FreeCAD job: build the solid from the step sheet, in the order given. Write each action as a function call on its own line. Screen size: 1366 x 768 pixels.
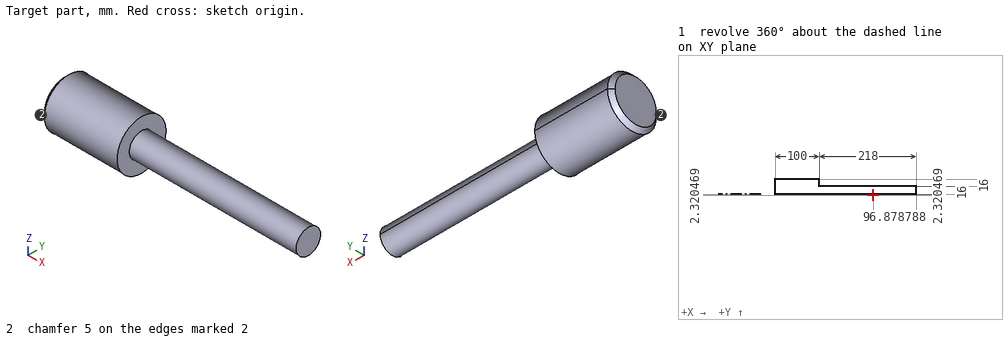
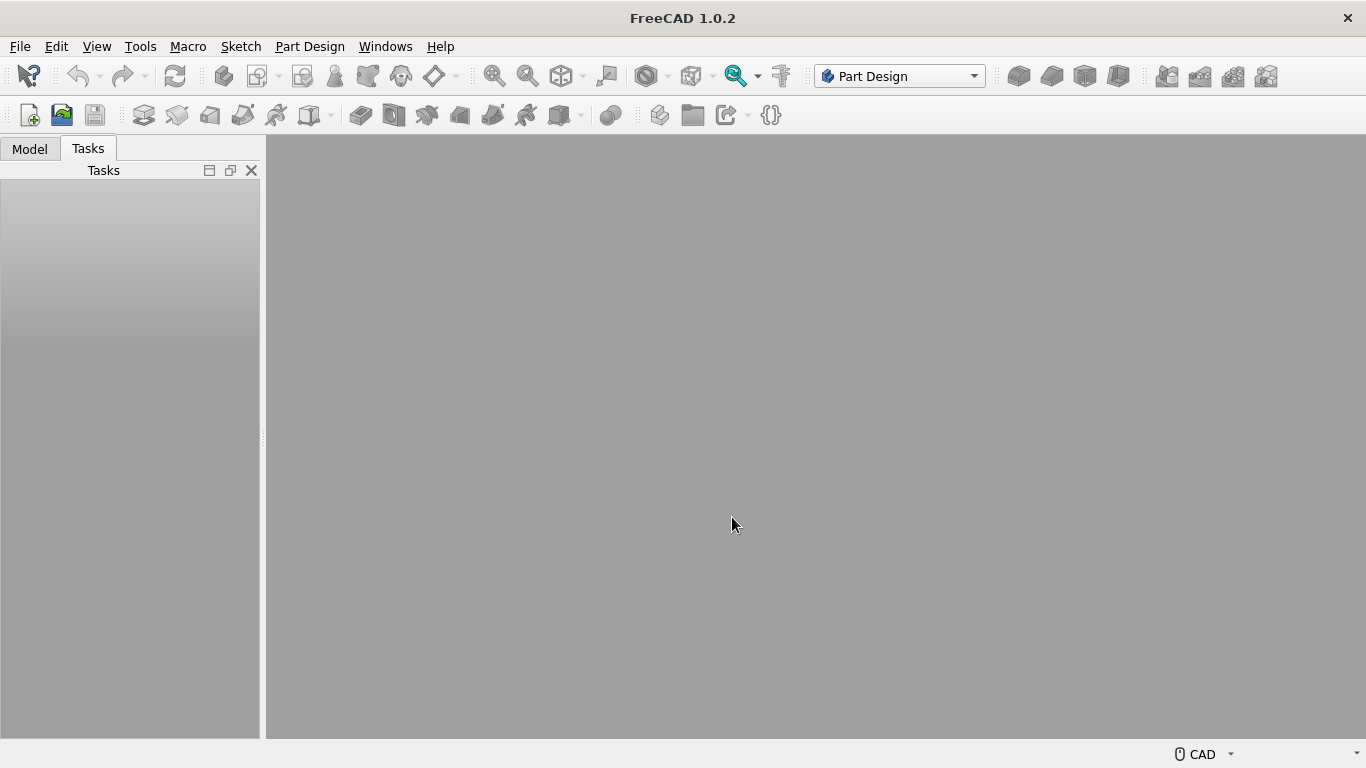
click(29, 116)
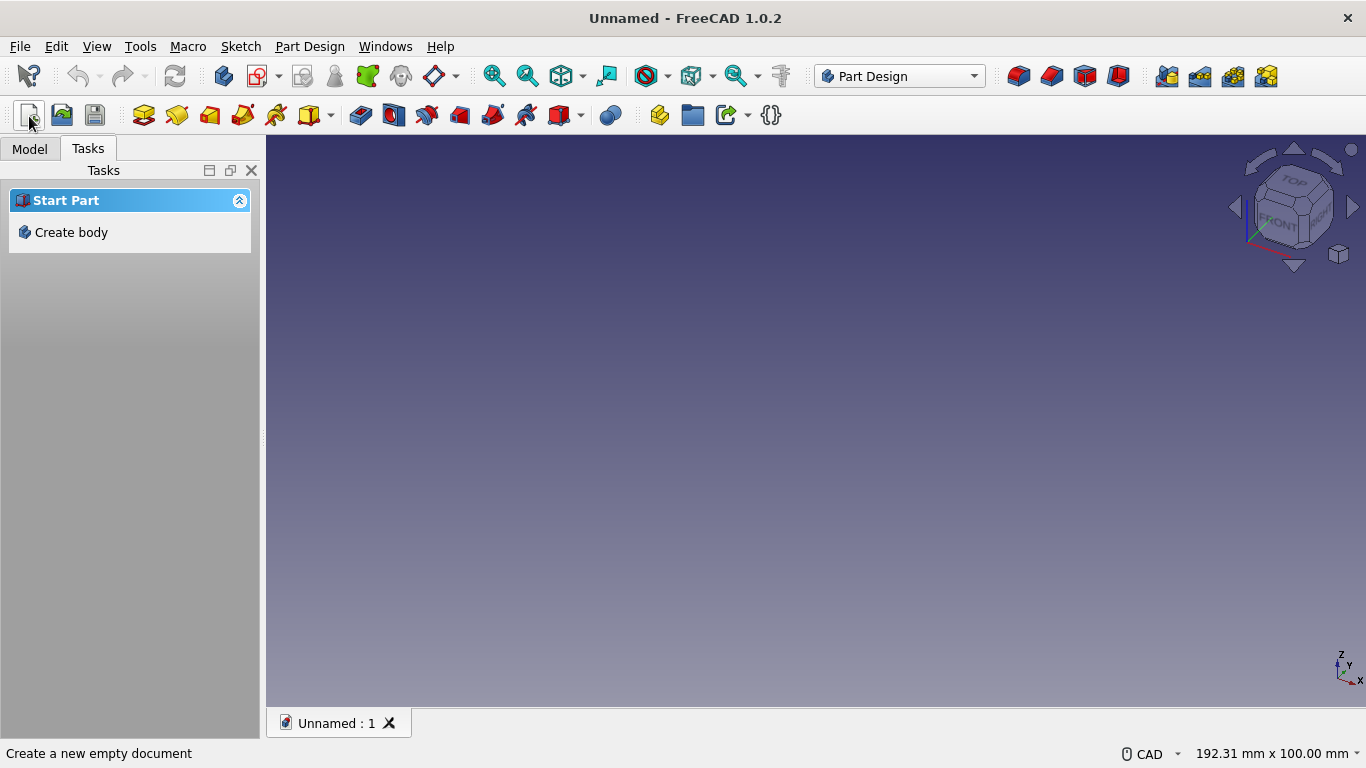
click(256, 76)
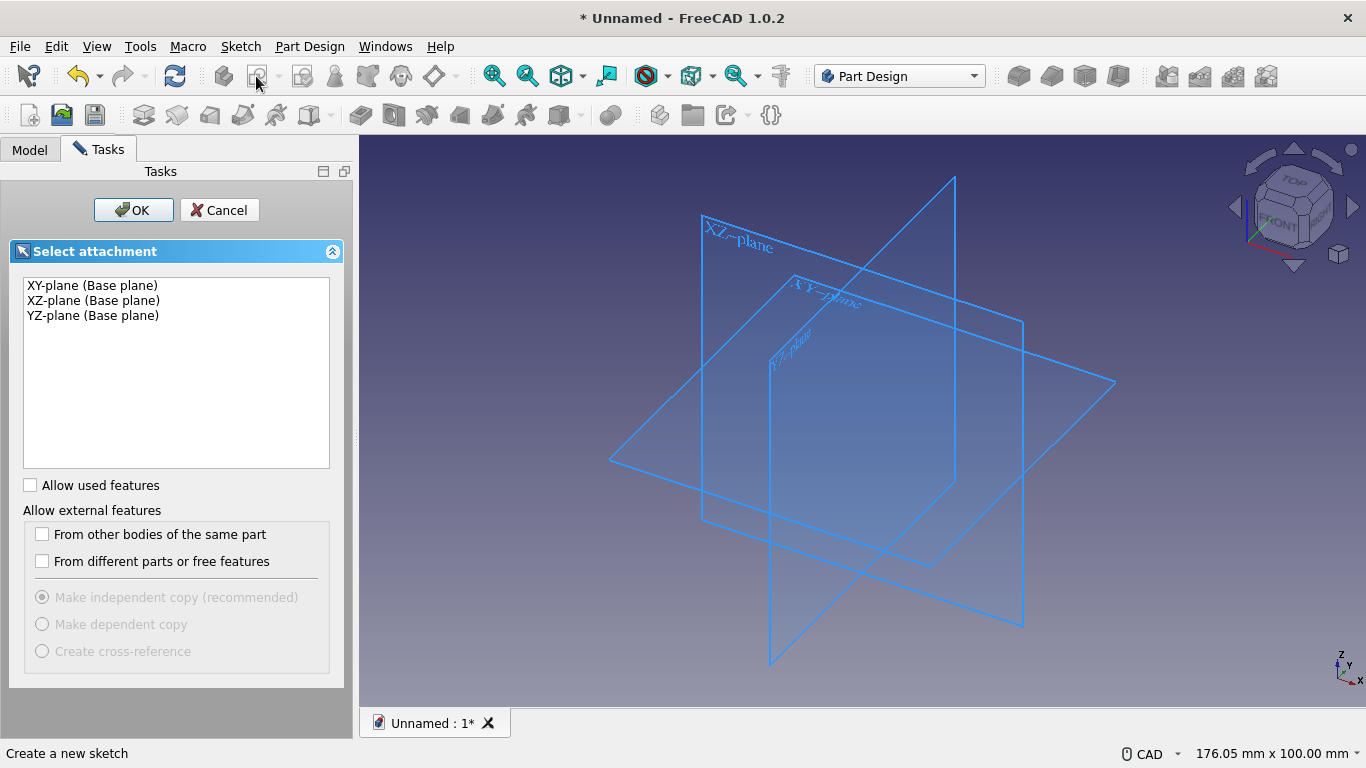
click(84, 286)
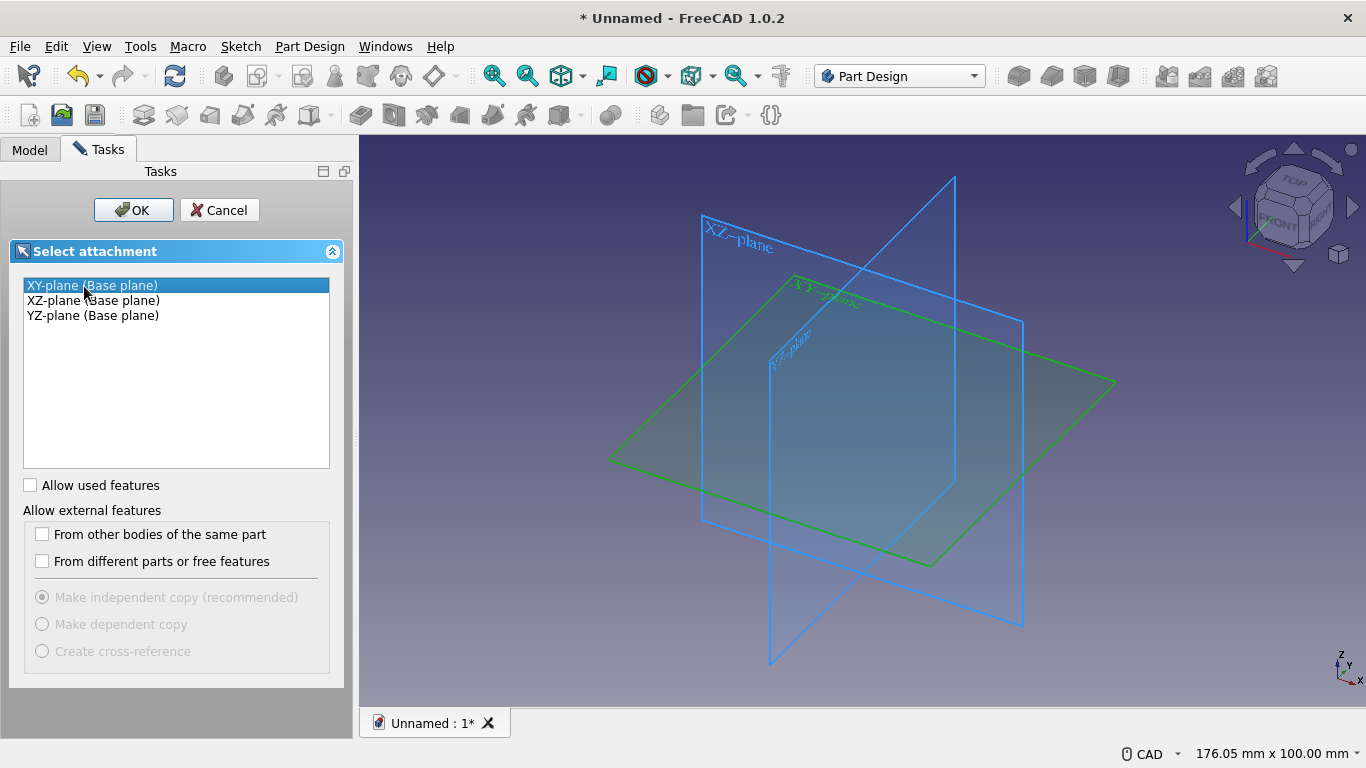
click(134, 210)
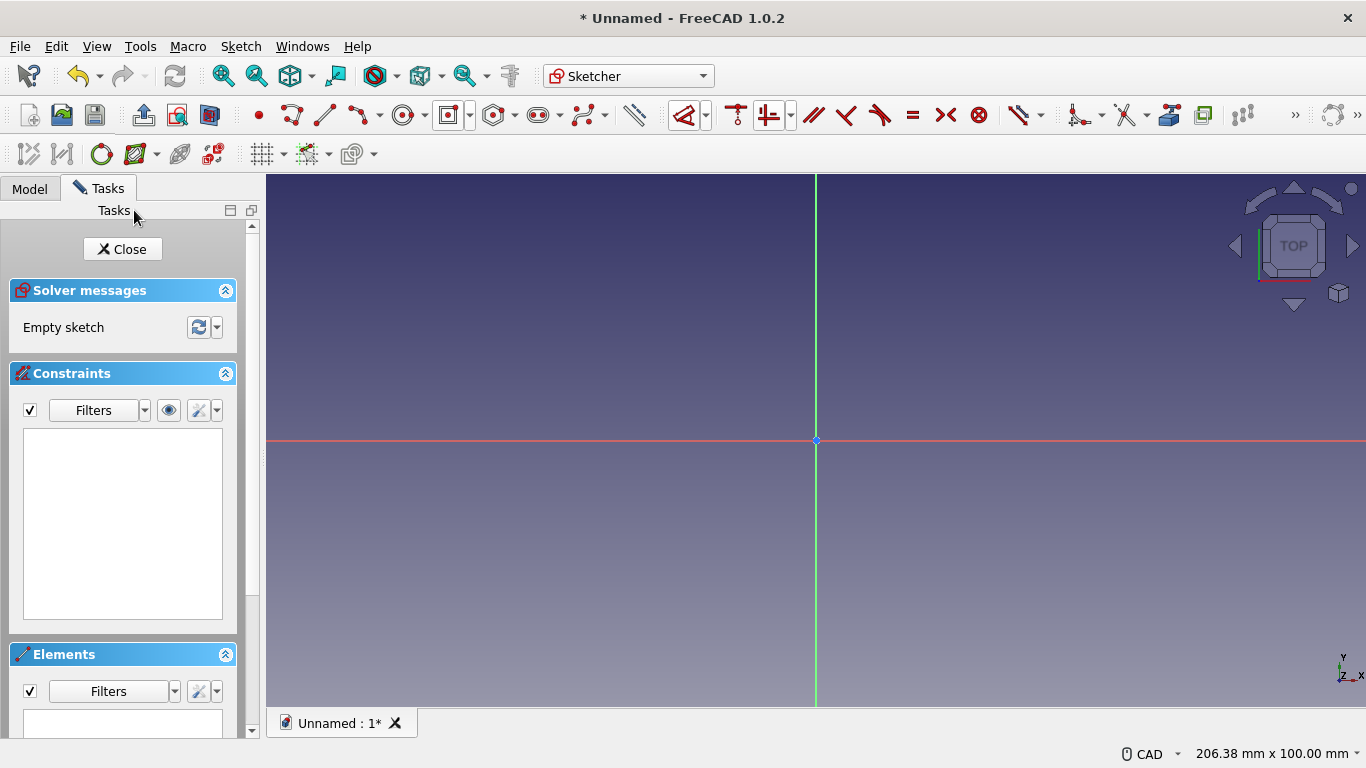
scroll(944, 470, down, 7)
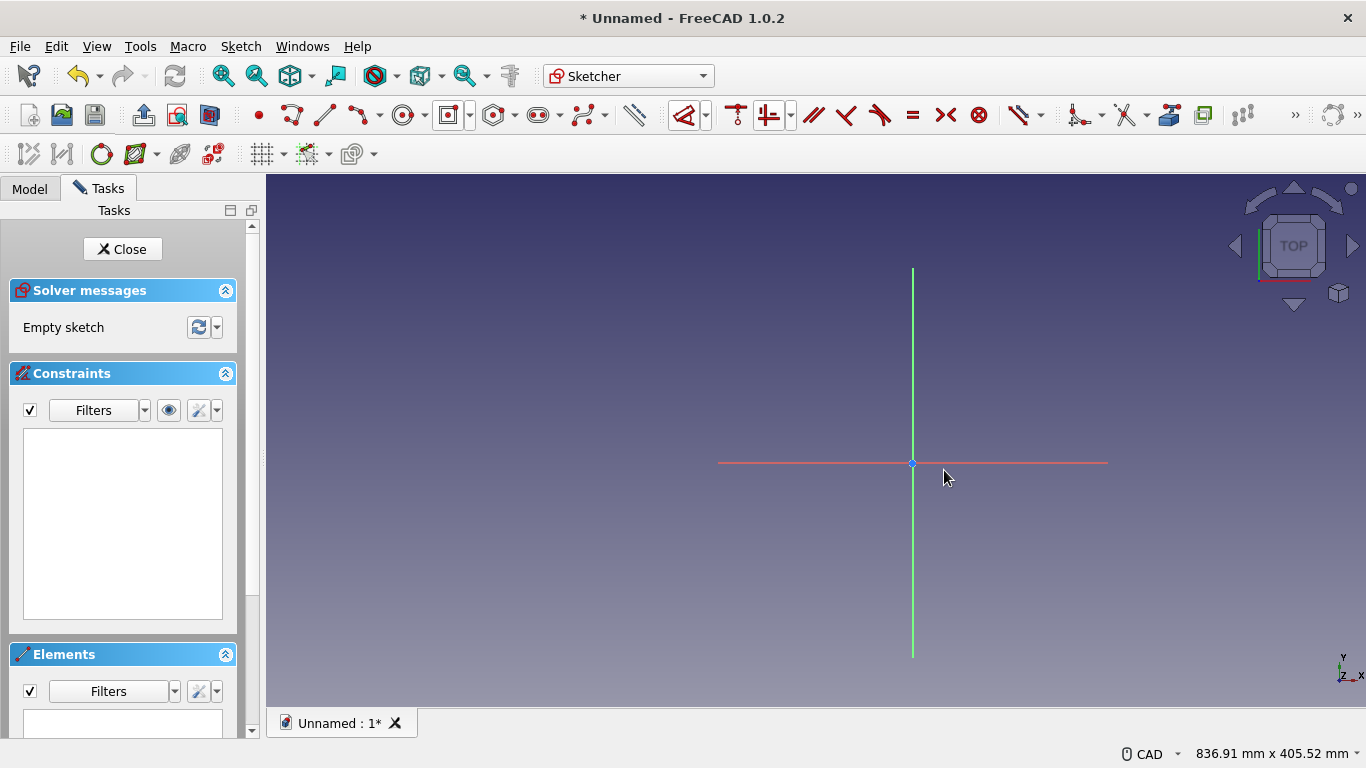
click(292, 116)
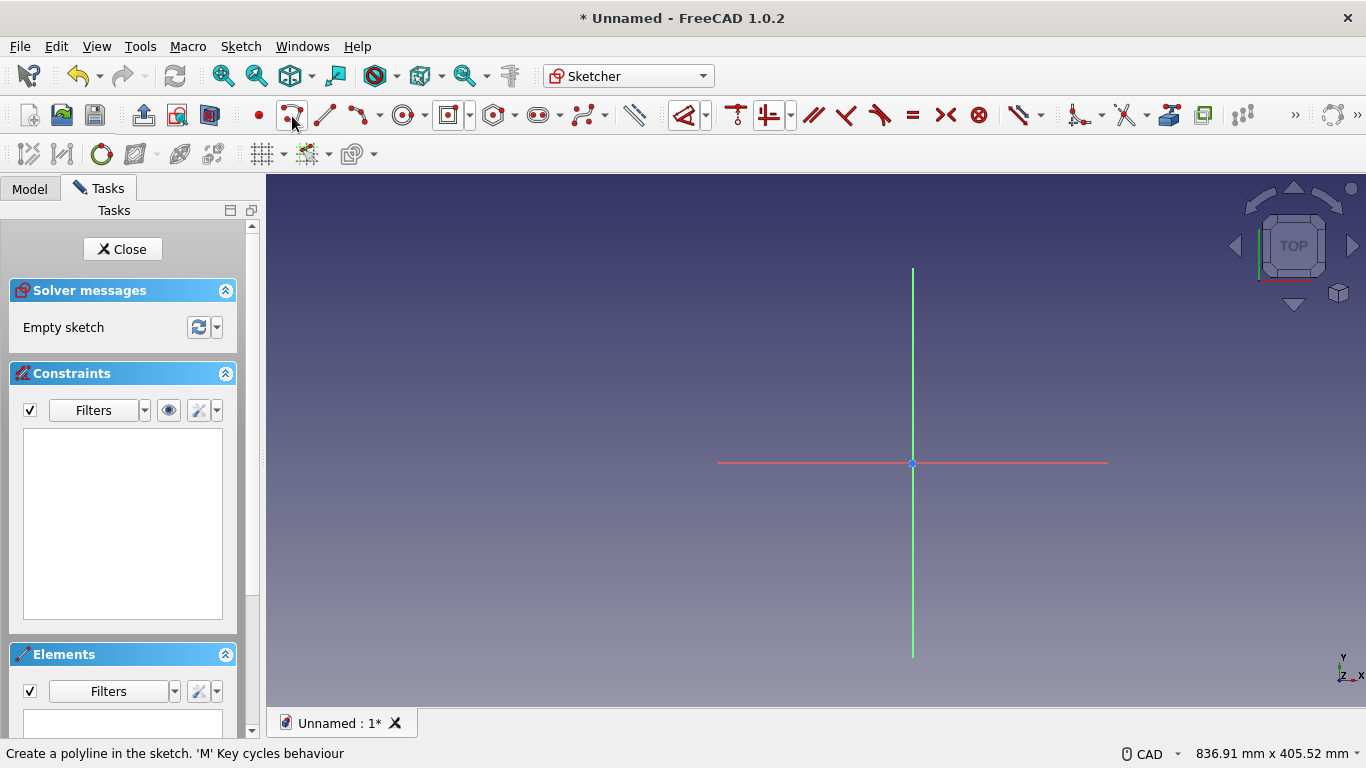
scroll(1040, 460, up, 9)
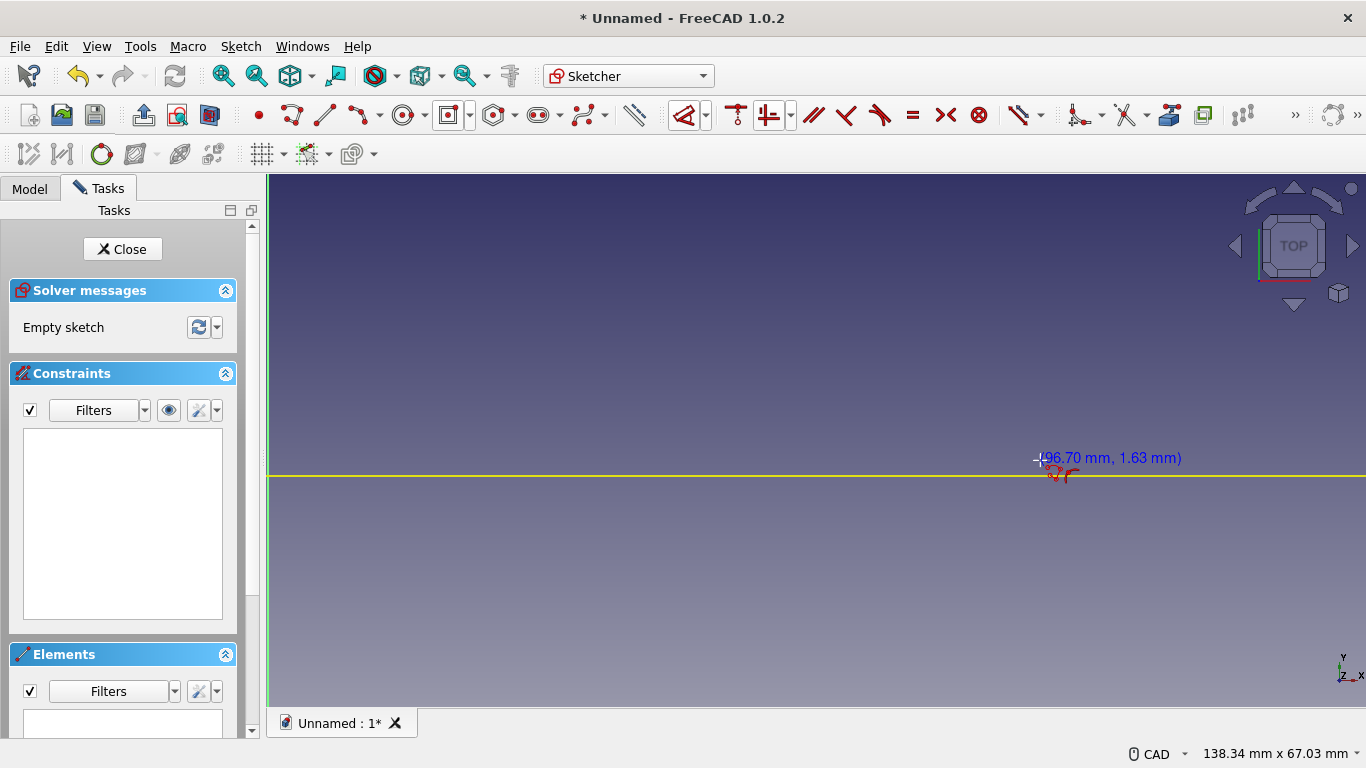
click(1038, 458)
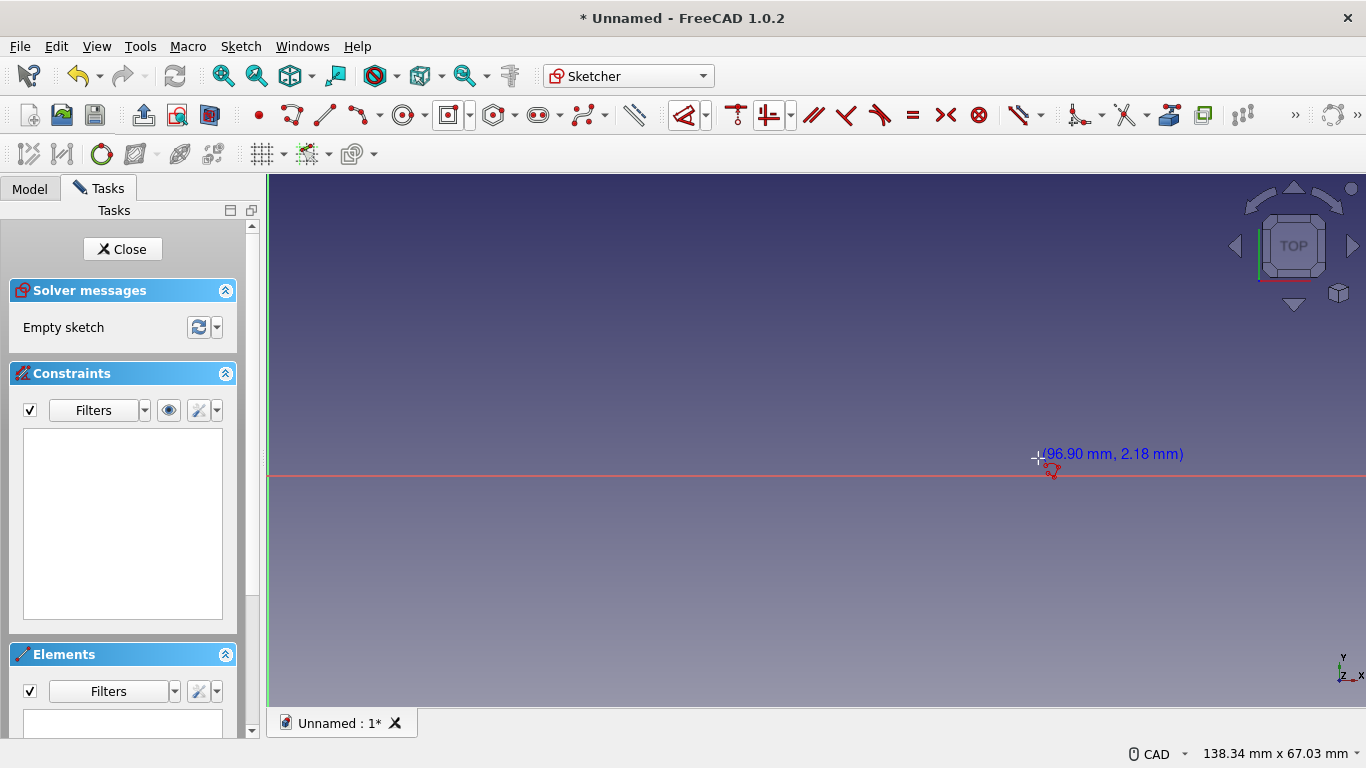
scroll(1041, 460, down, 9)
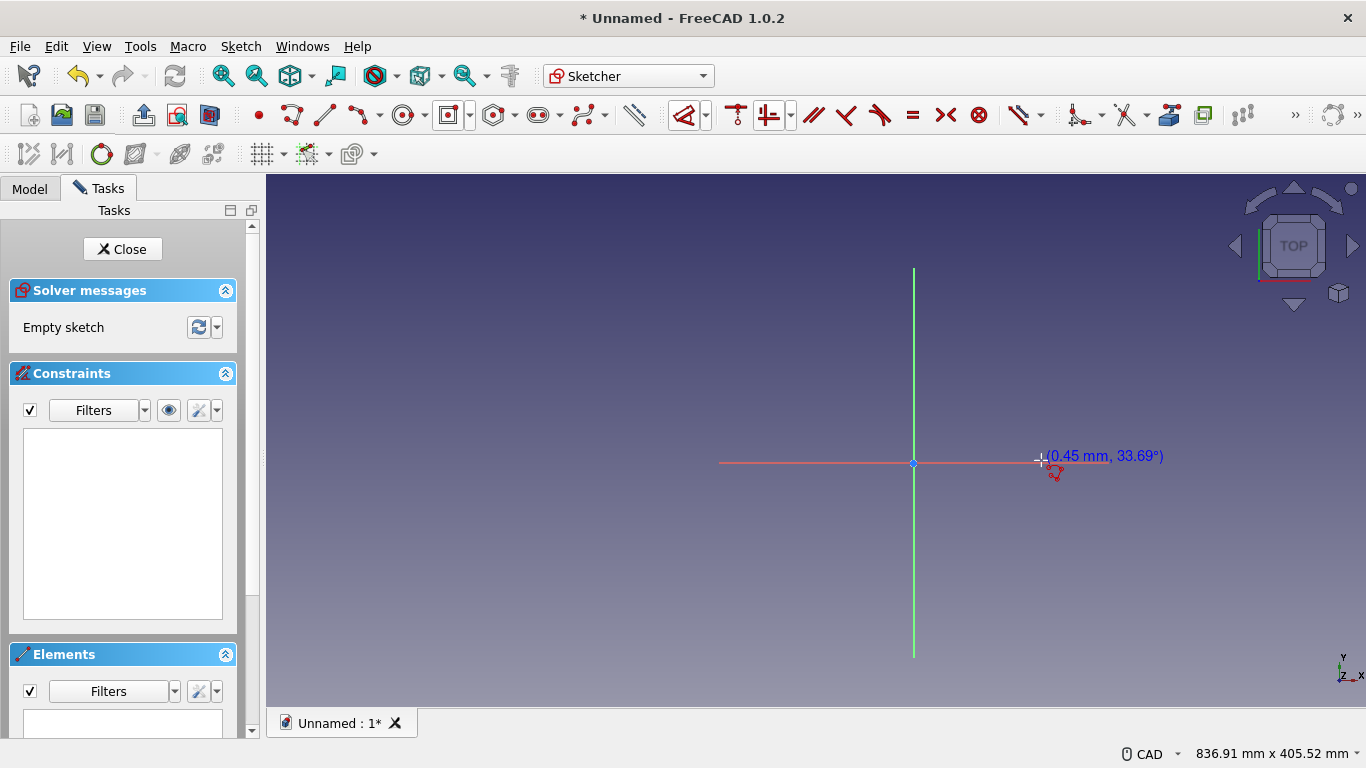
click(1041, 439)
click(755, 439)
click(755, 418)
click(623, 418)